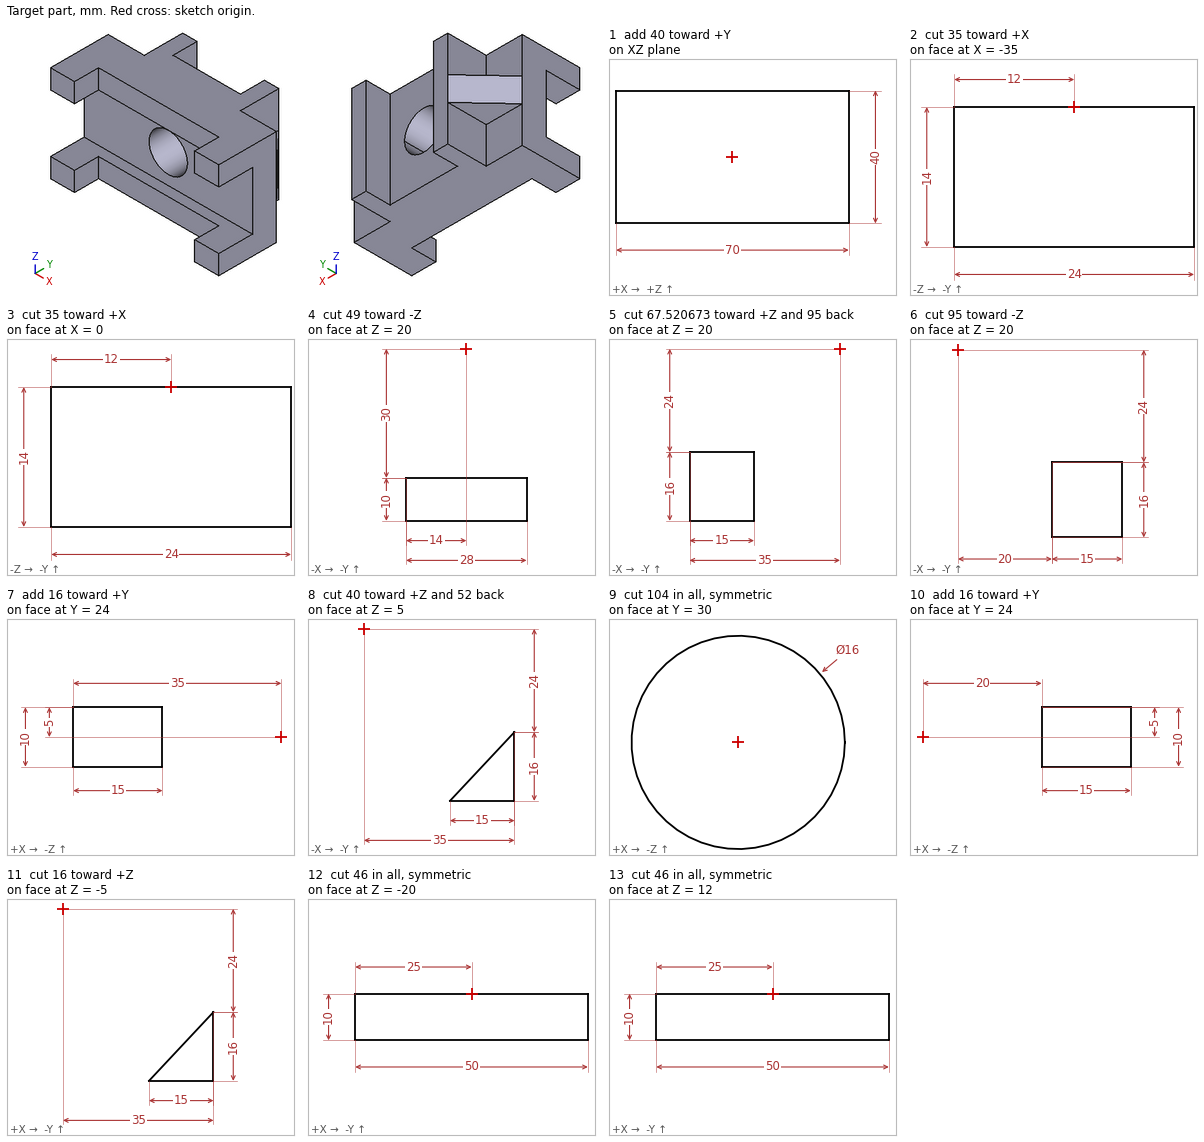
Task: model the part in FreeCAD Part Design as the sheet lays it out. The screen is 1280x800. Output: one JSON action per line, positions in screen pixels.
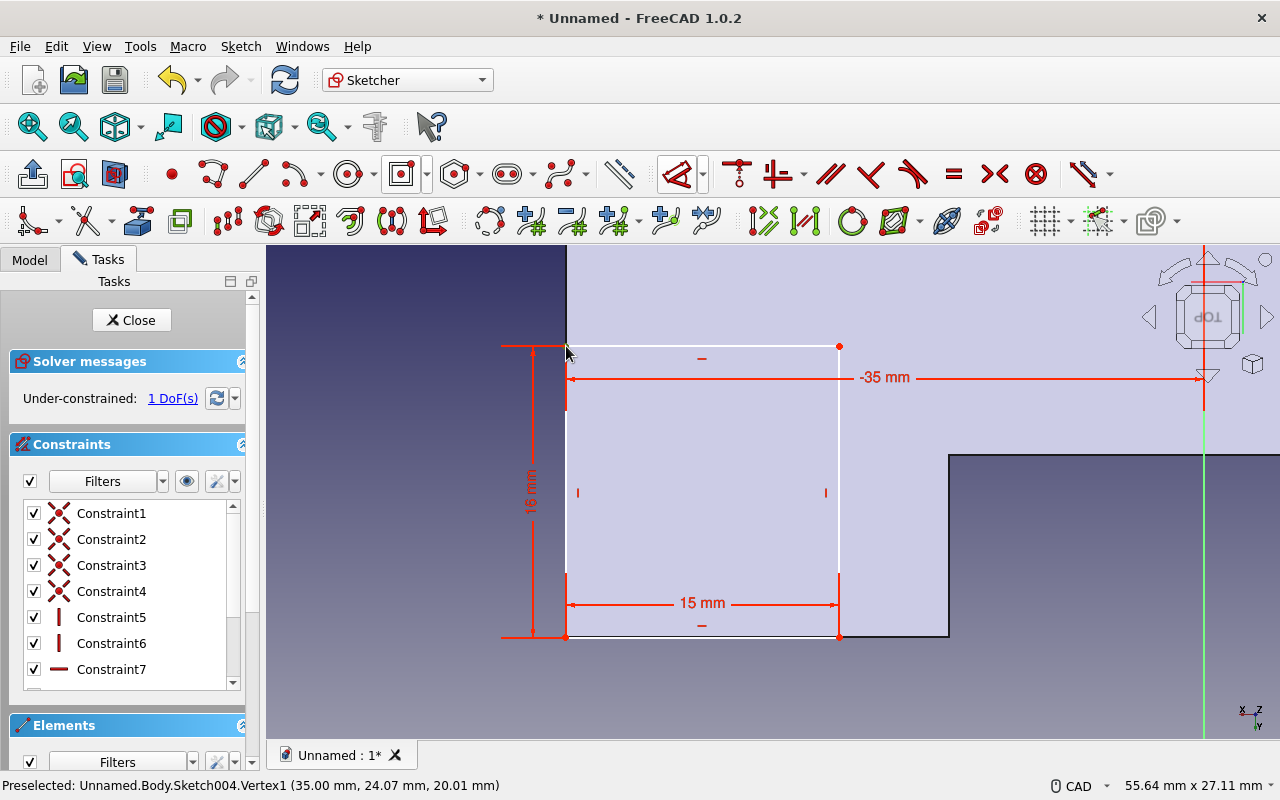
{"action": "key", "text": "i"}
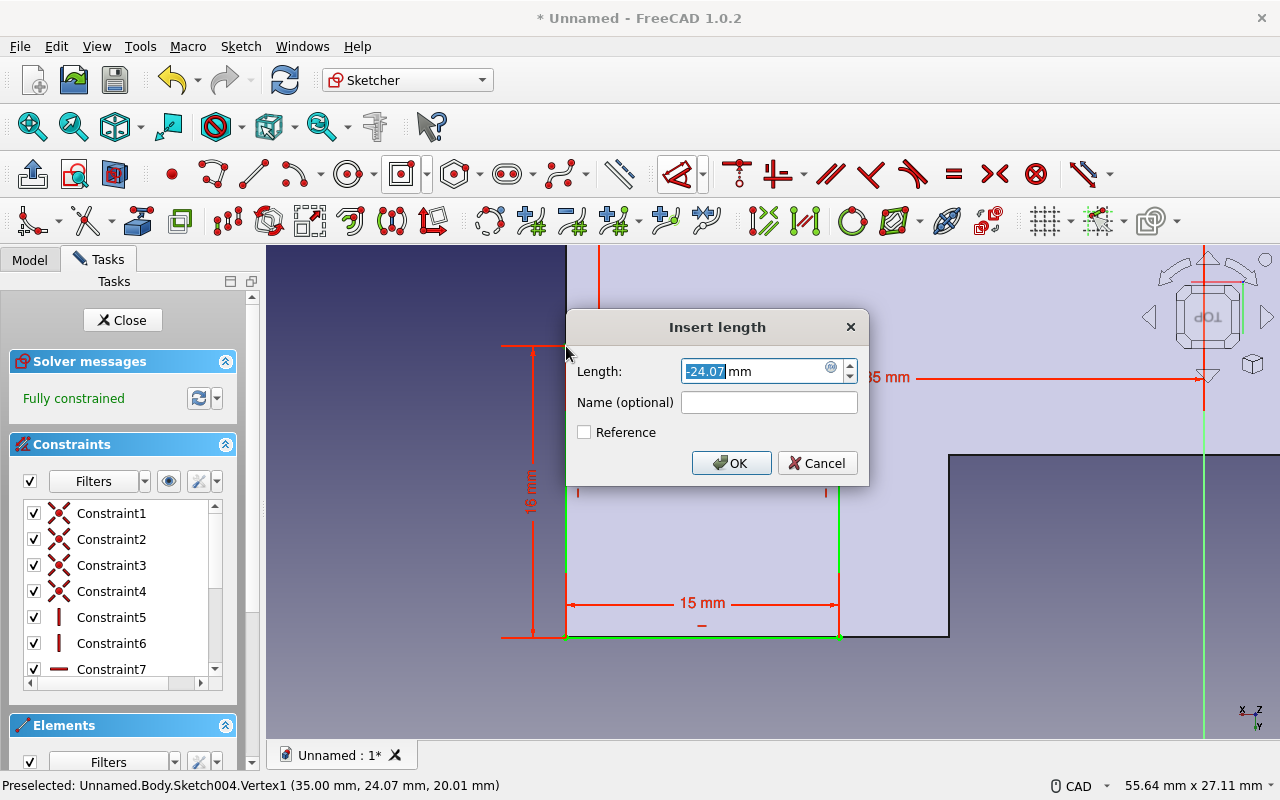
{"action": "type", "text": "-24"}
{"action": "key", "text": "Return"}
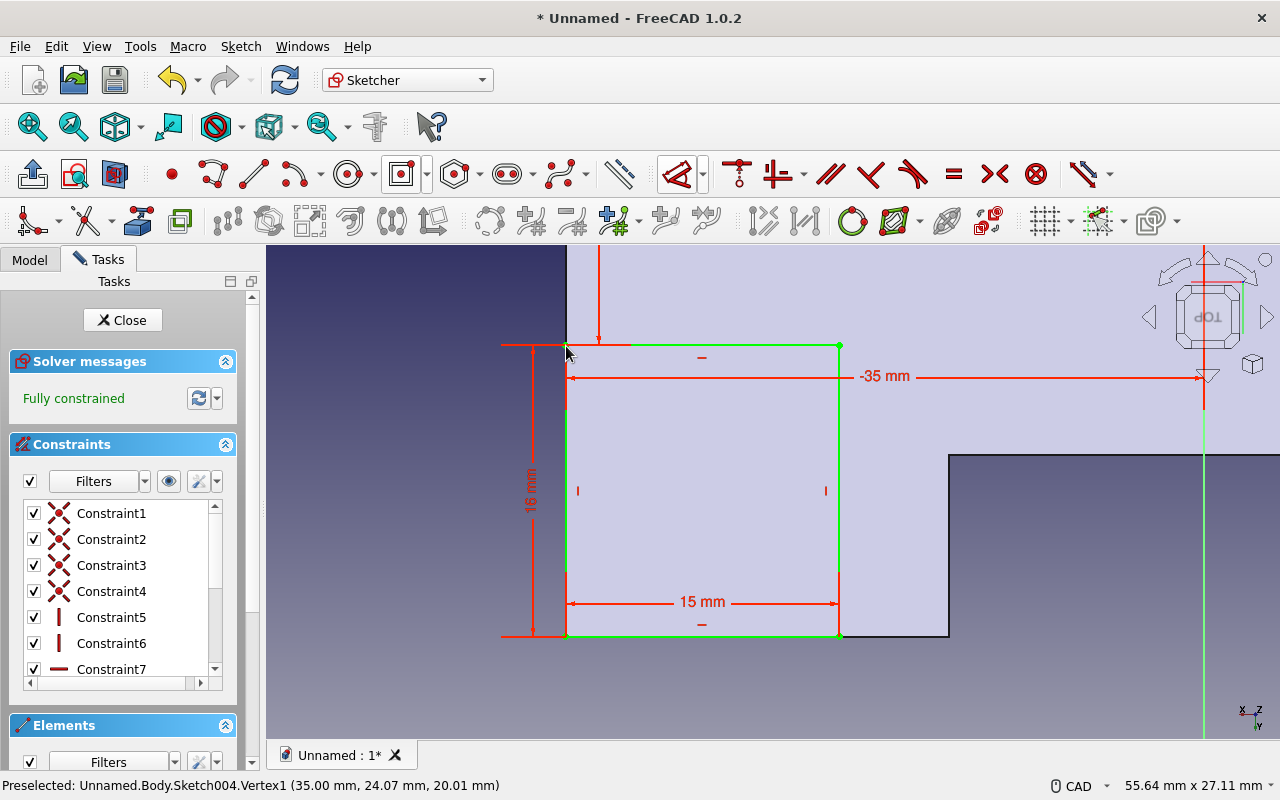
{"action": "left_click", "coordinate": [123, 320]}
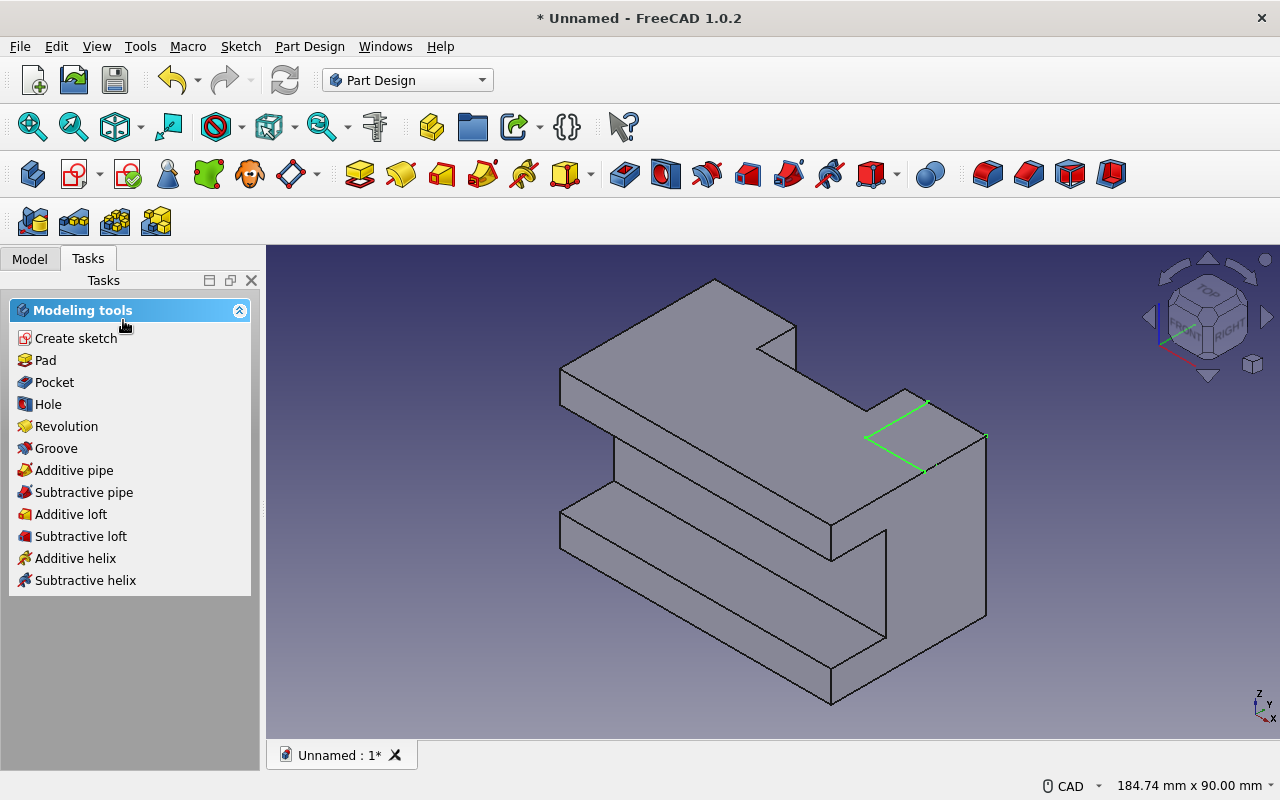
{"action": "left_click", "coordinate": [625, 174]}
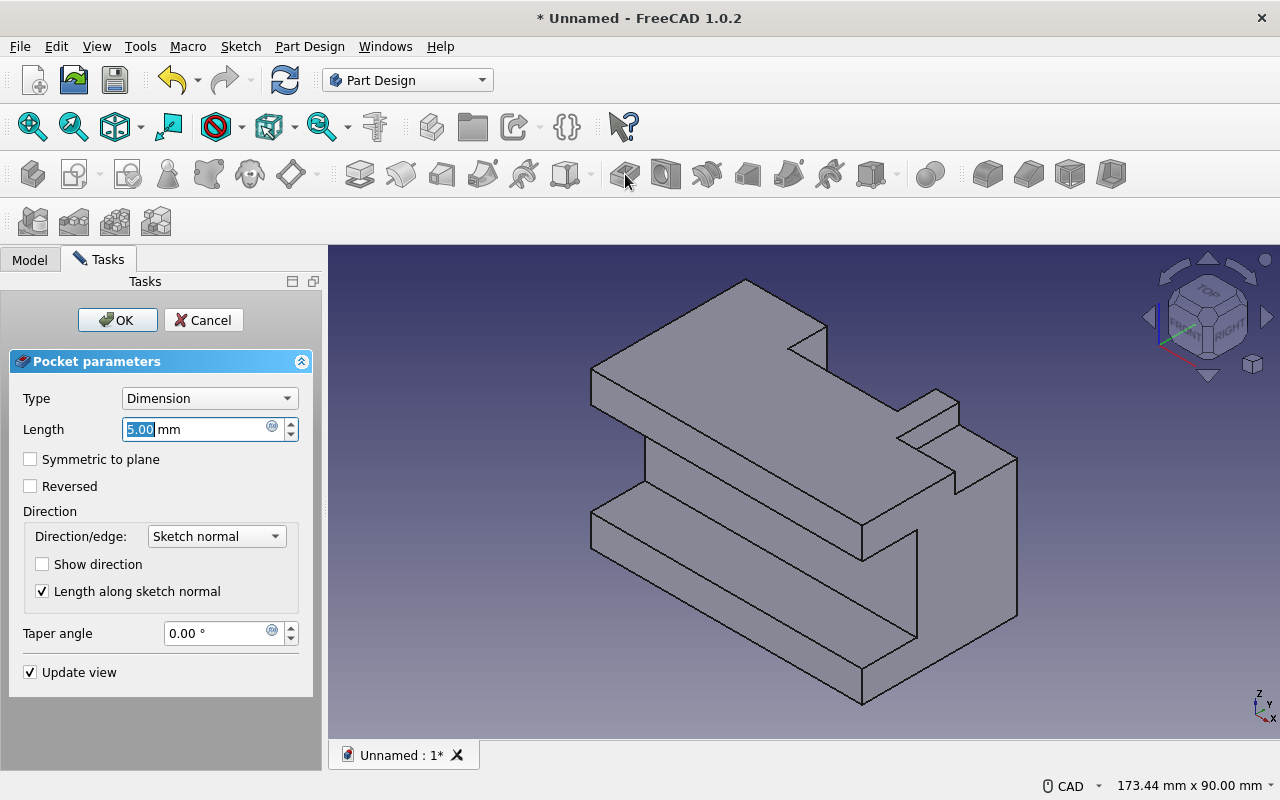
{"action": "left_click", "coordinate": [210, 398]}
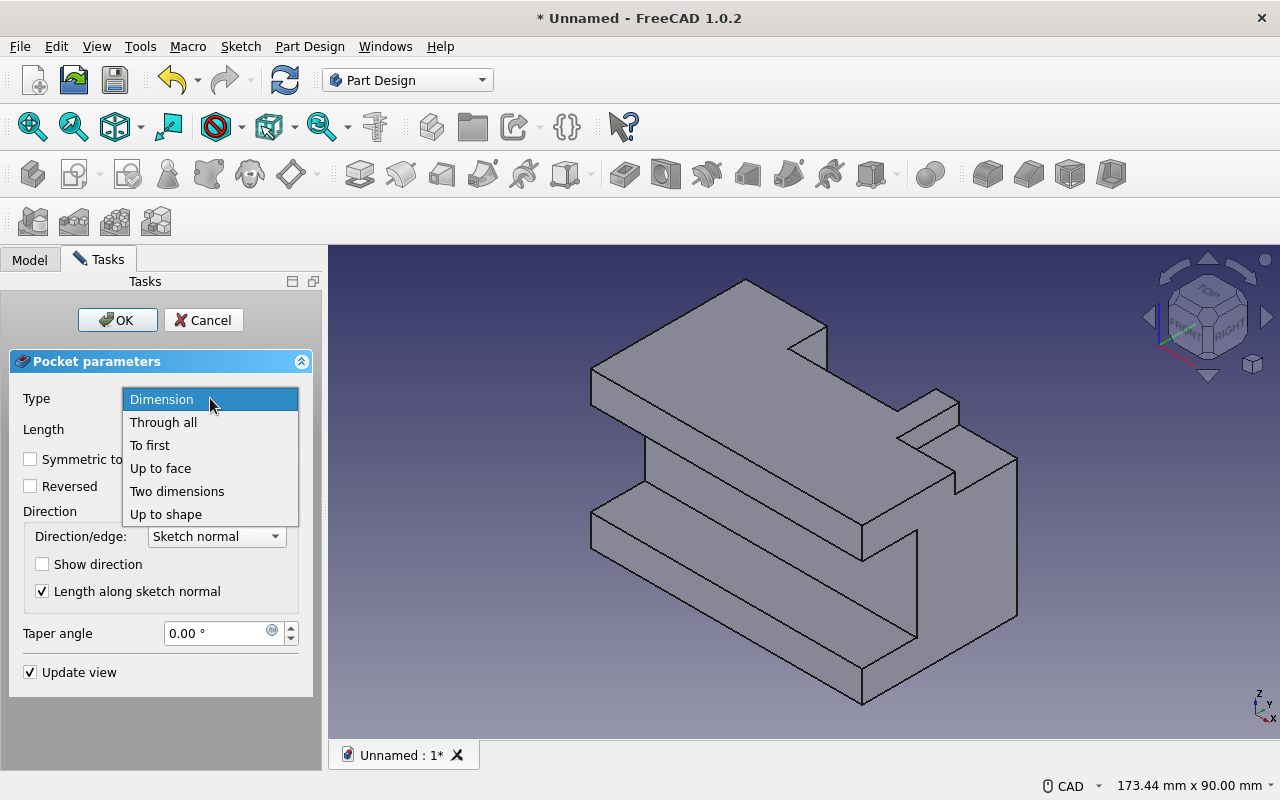
{"action": "left_click", "coordinate": [208, 492]}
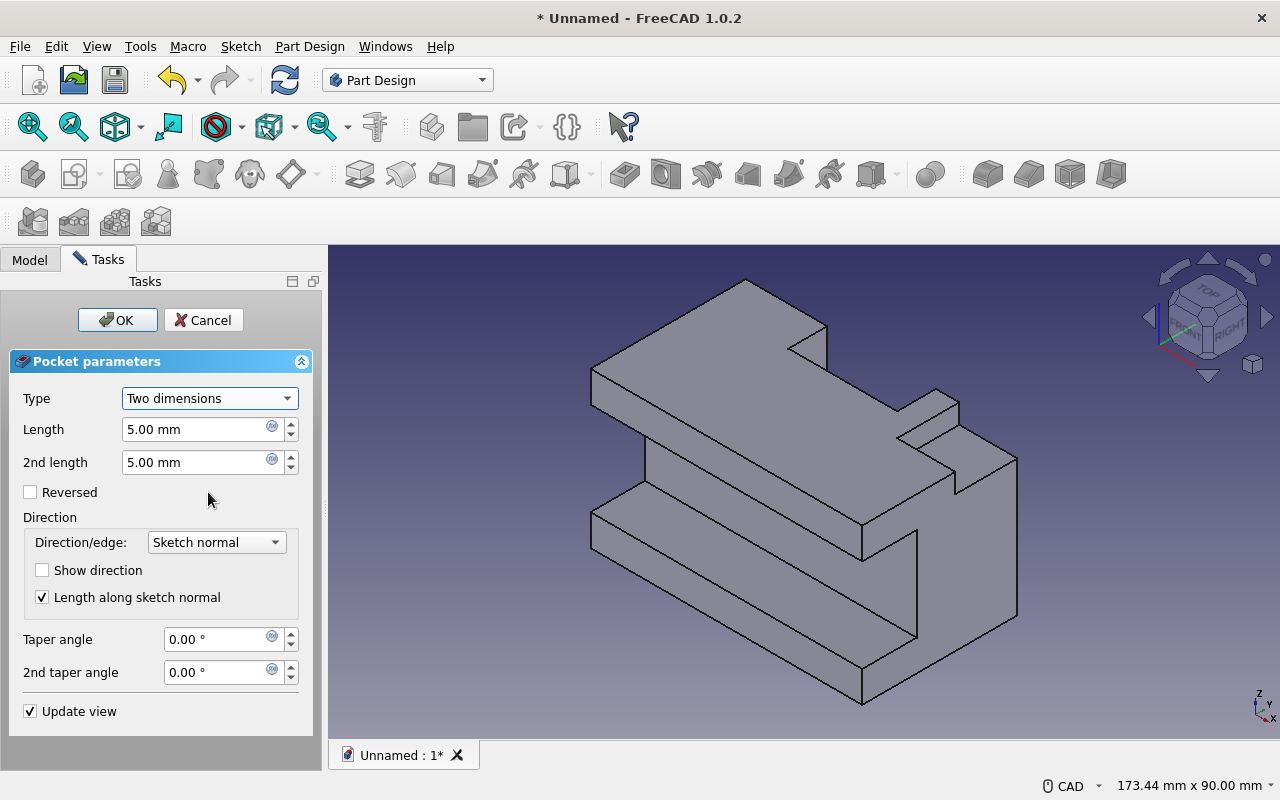
{"action": "triple_click", "coordinate": [204, 430]}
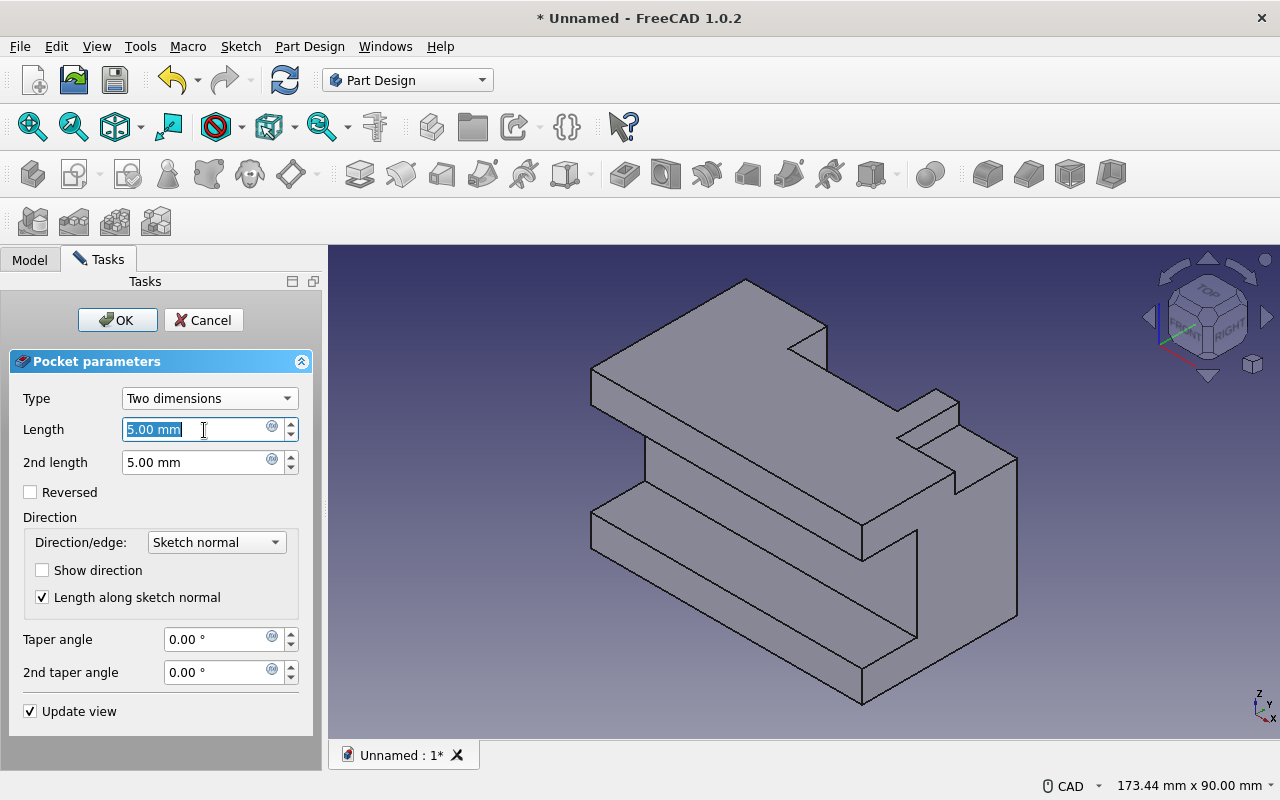
{"action": "type", "text": "67.520673"}
{"action": "key", "text": "Tab"}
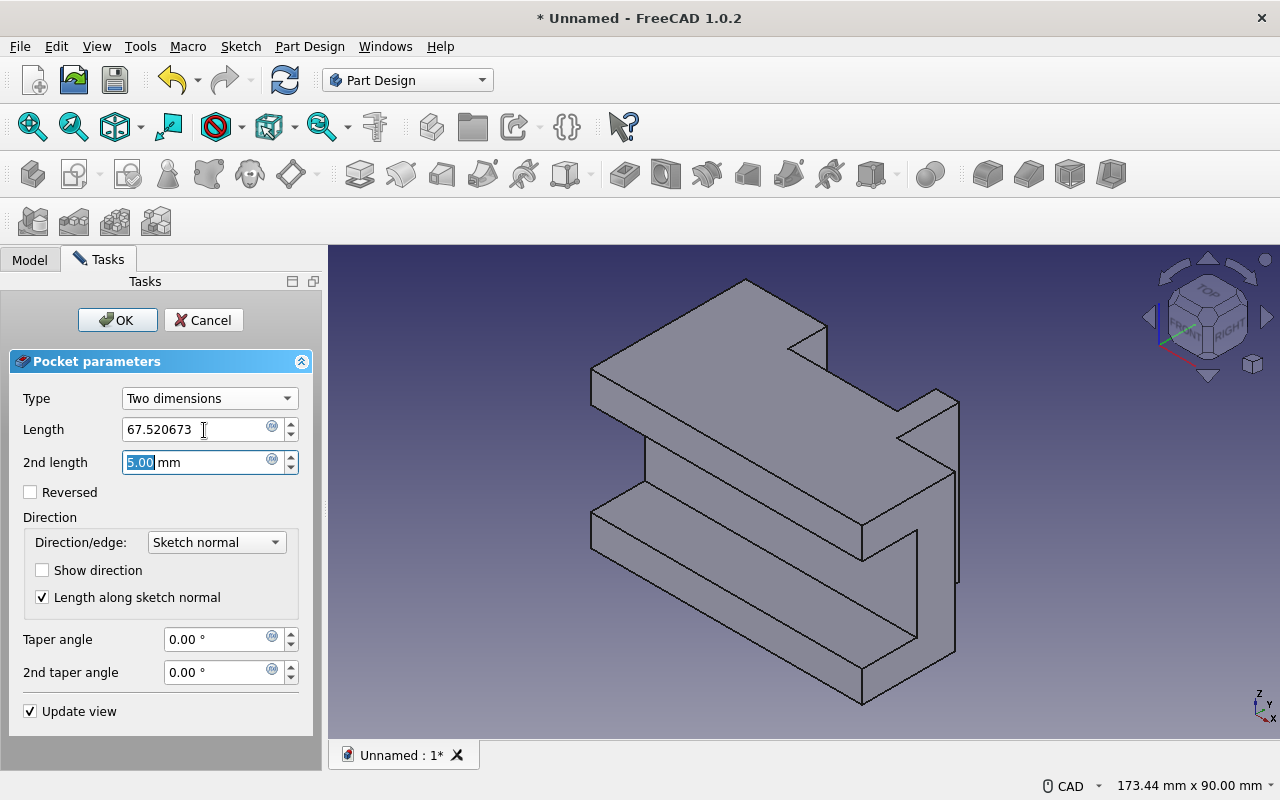
{"action": "type", "text": "95"}
{"action": "key", "text": "Tab"}